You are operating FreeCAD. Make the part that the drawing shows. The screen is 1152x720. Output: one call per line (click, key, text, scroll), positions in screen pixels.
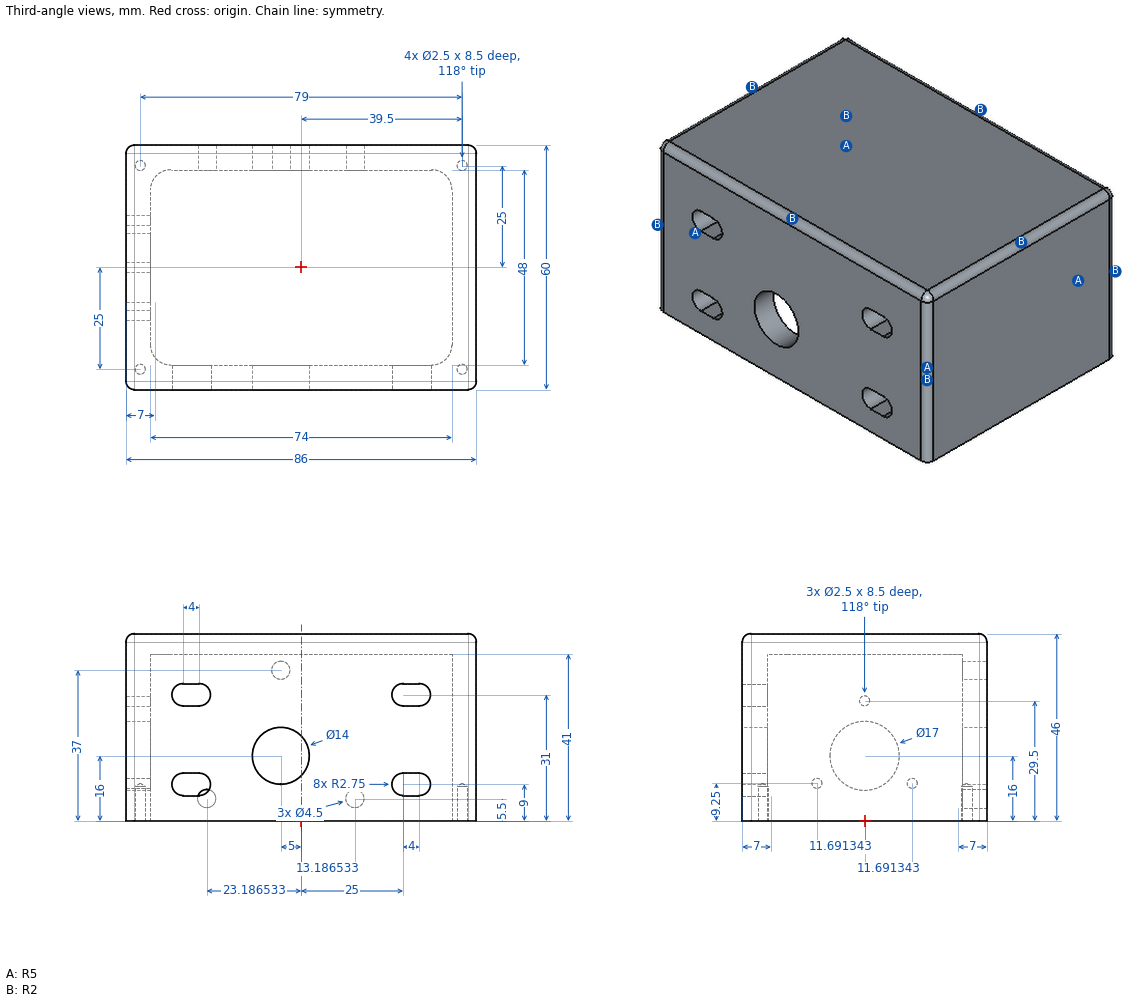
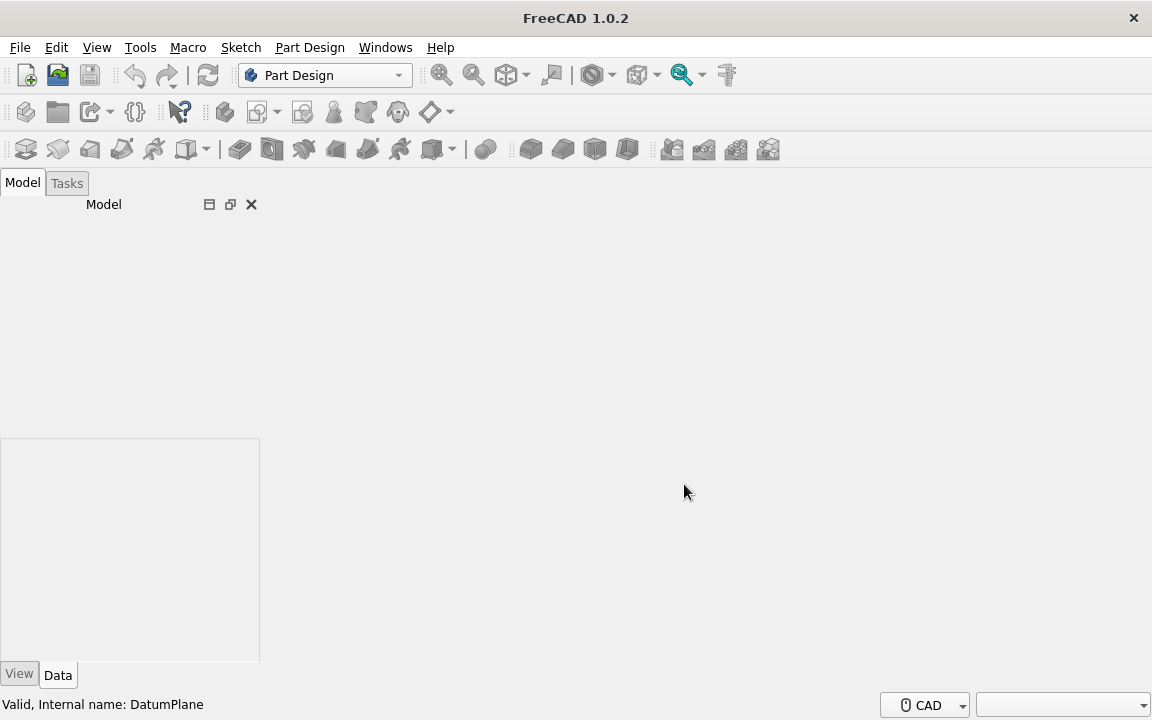
key(ctrl+n)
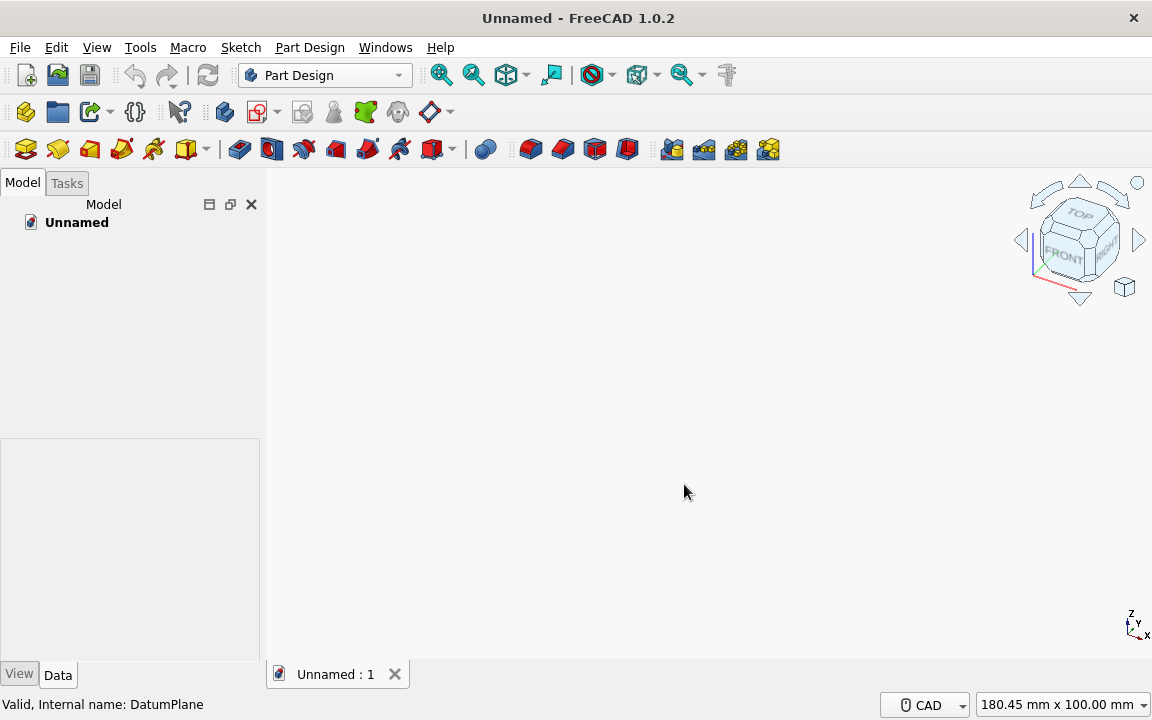
click(258, 112)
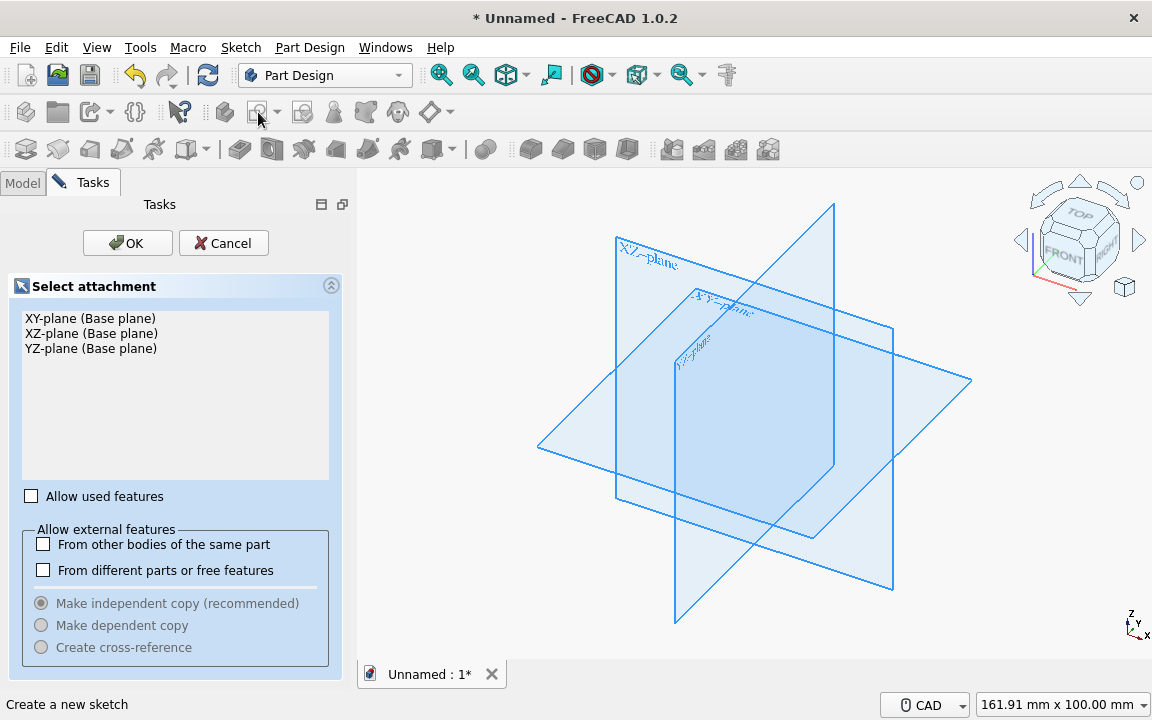
click(82, 318)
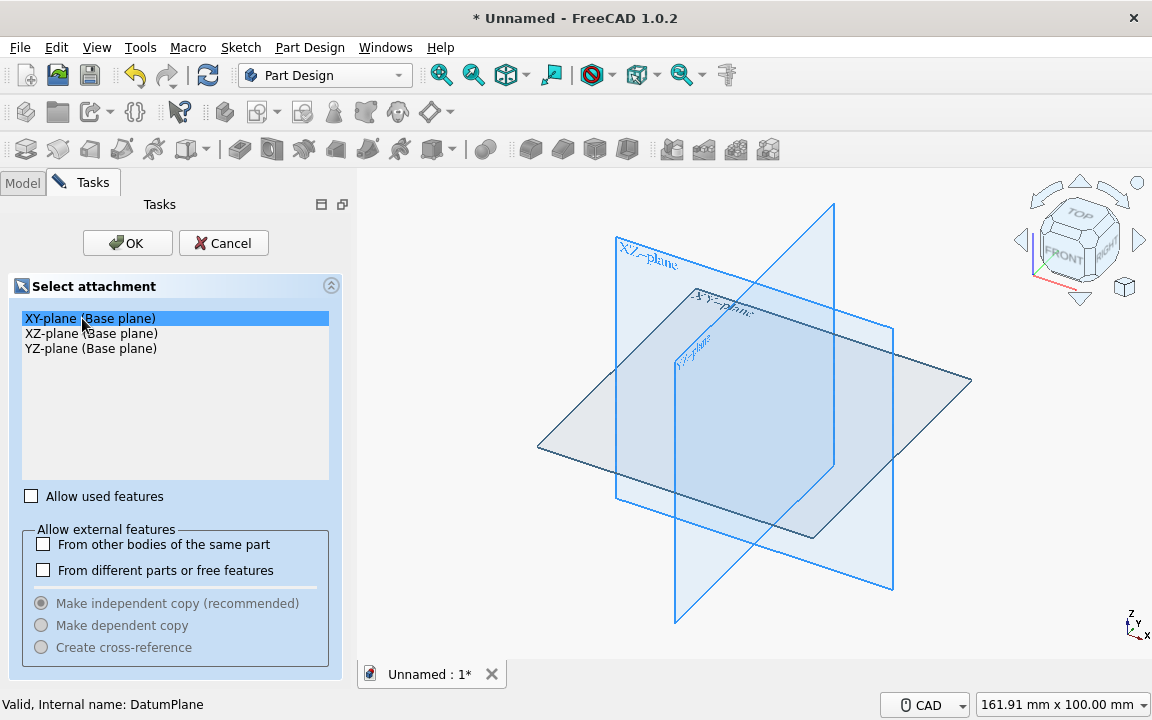
click(128, 243)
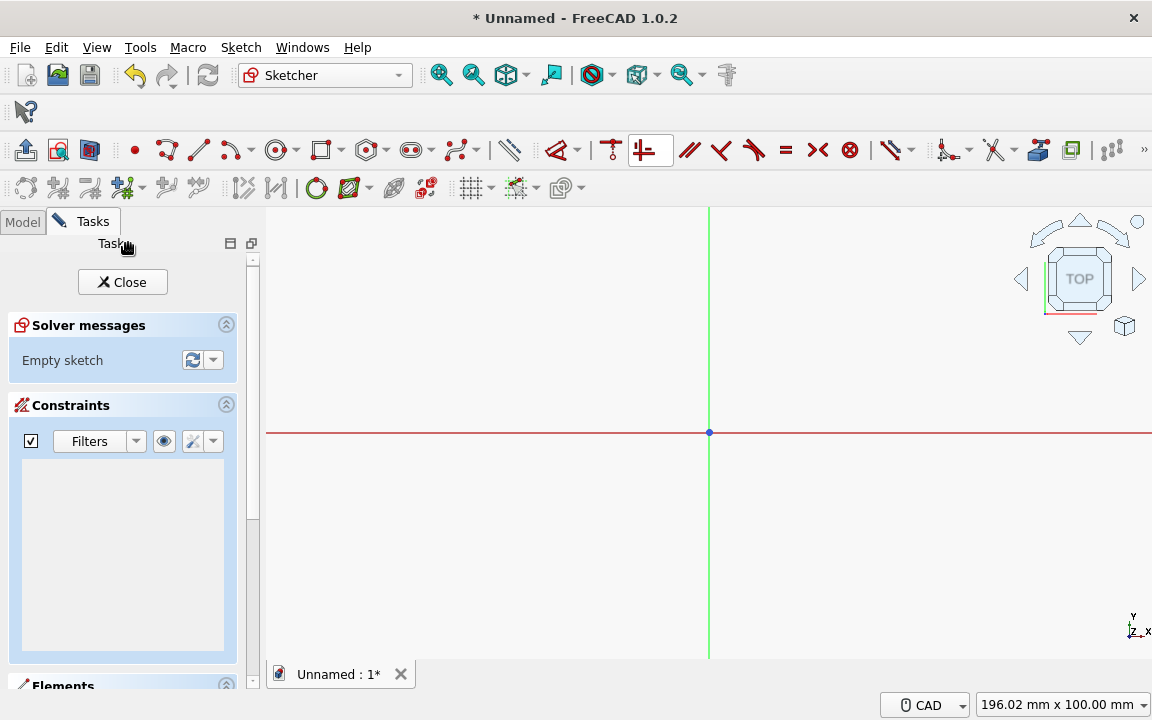
click(344, 150)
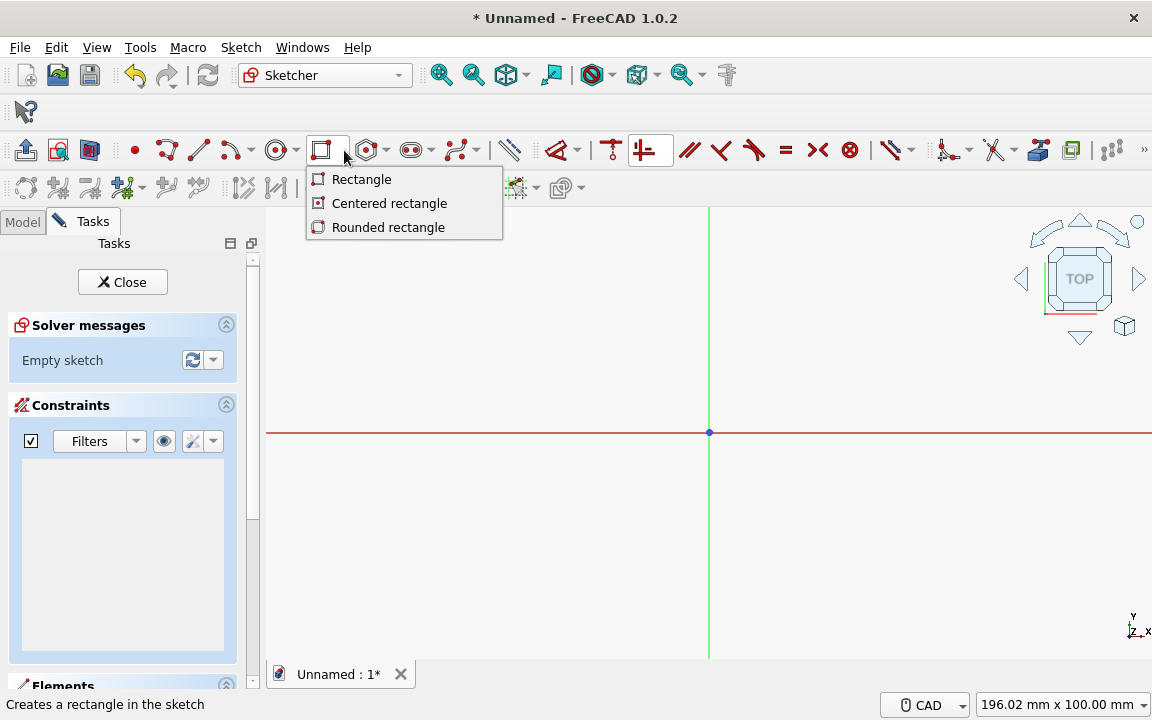
click(404, 203)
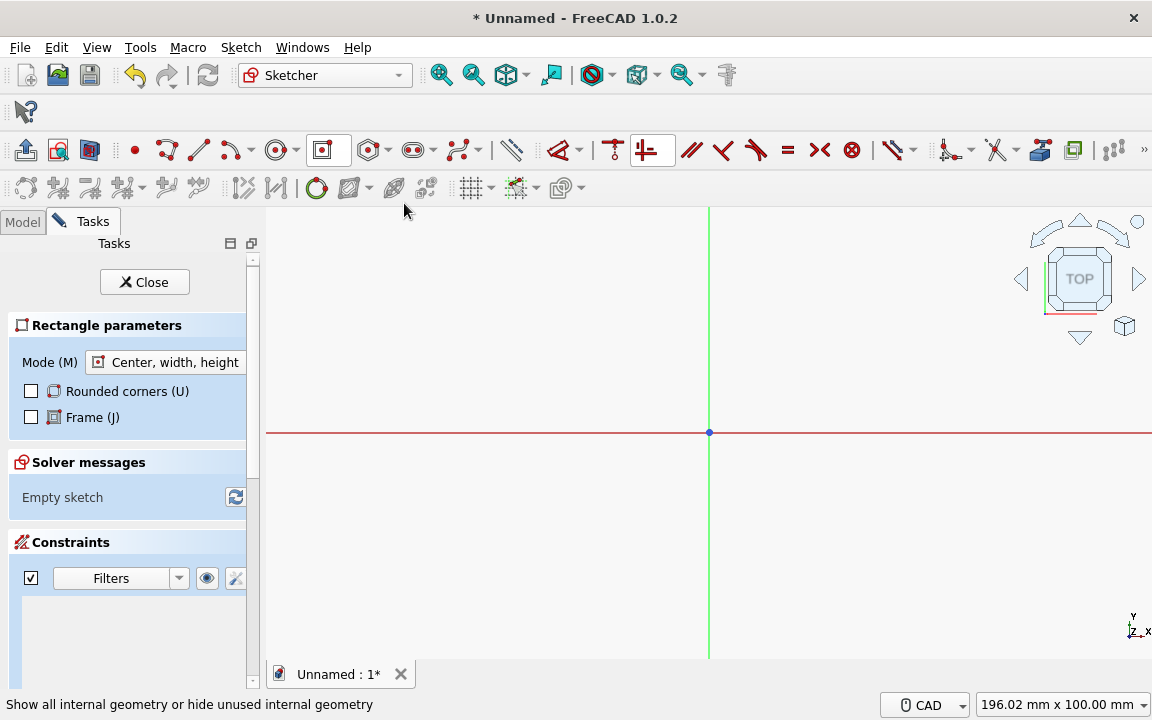
click(709, 433)
click(903, 297)
key(Escape)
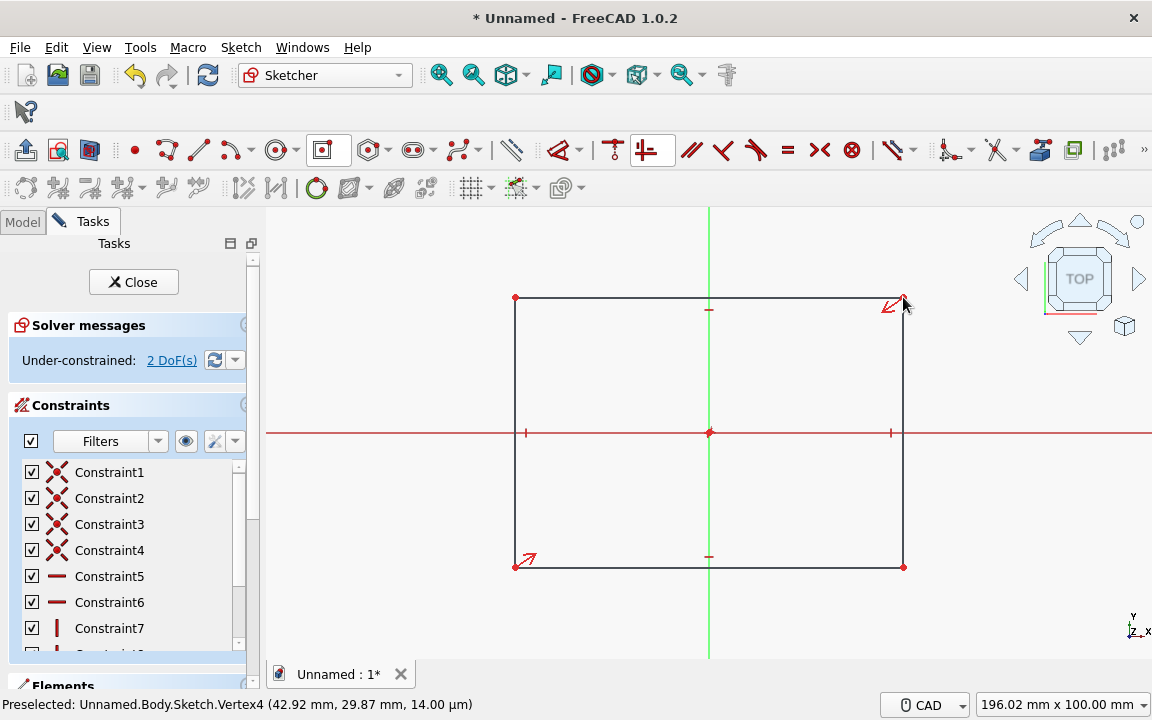
click(558, 150)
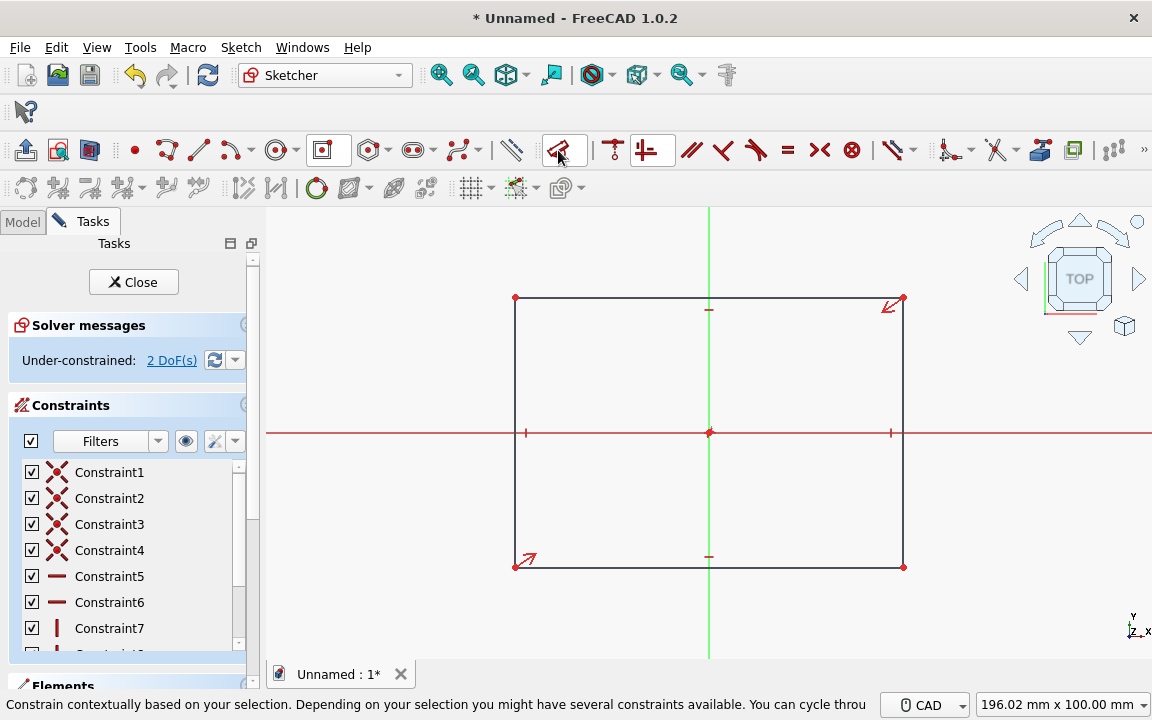
click(631, 568)
click(620, 602)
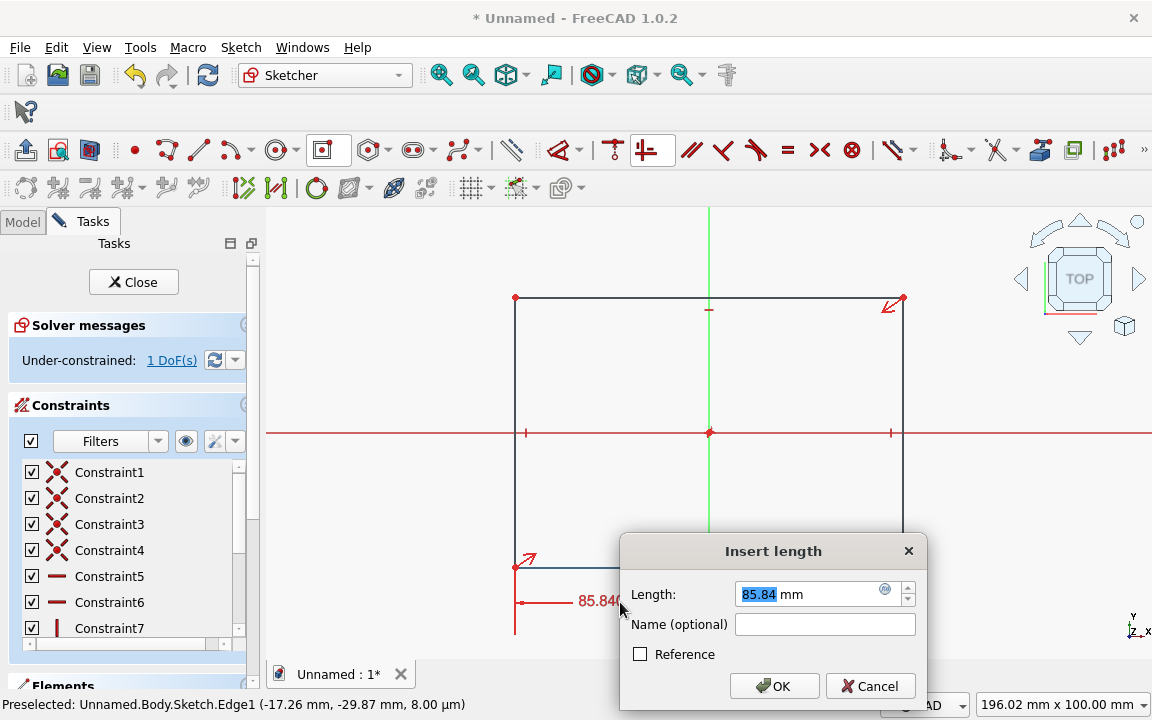
text(86)
key(Return)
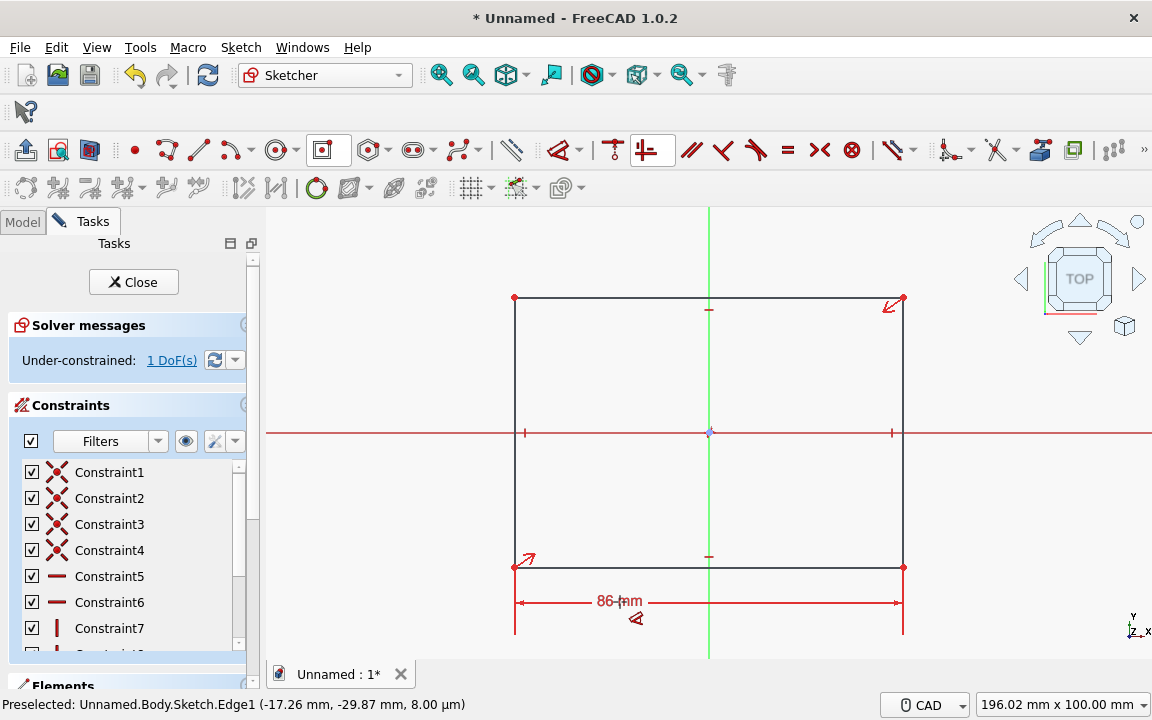
click(903, 487)
click(937, 371)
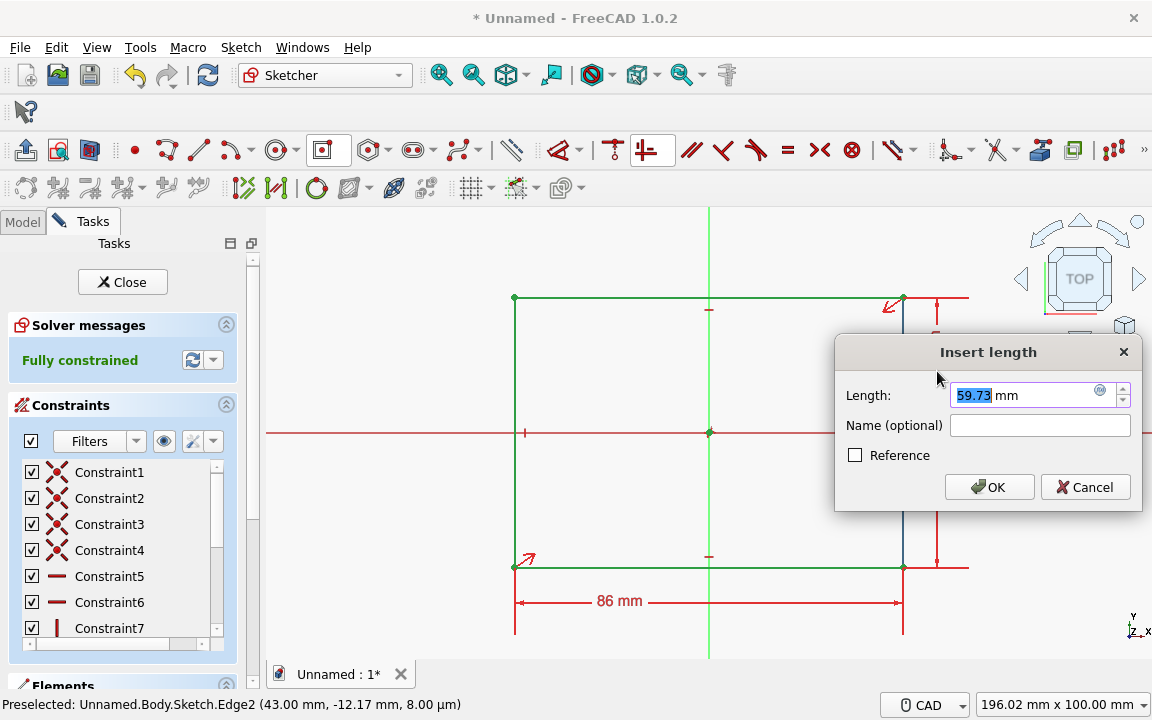
text(60)
key(Return)
key(Escape)